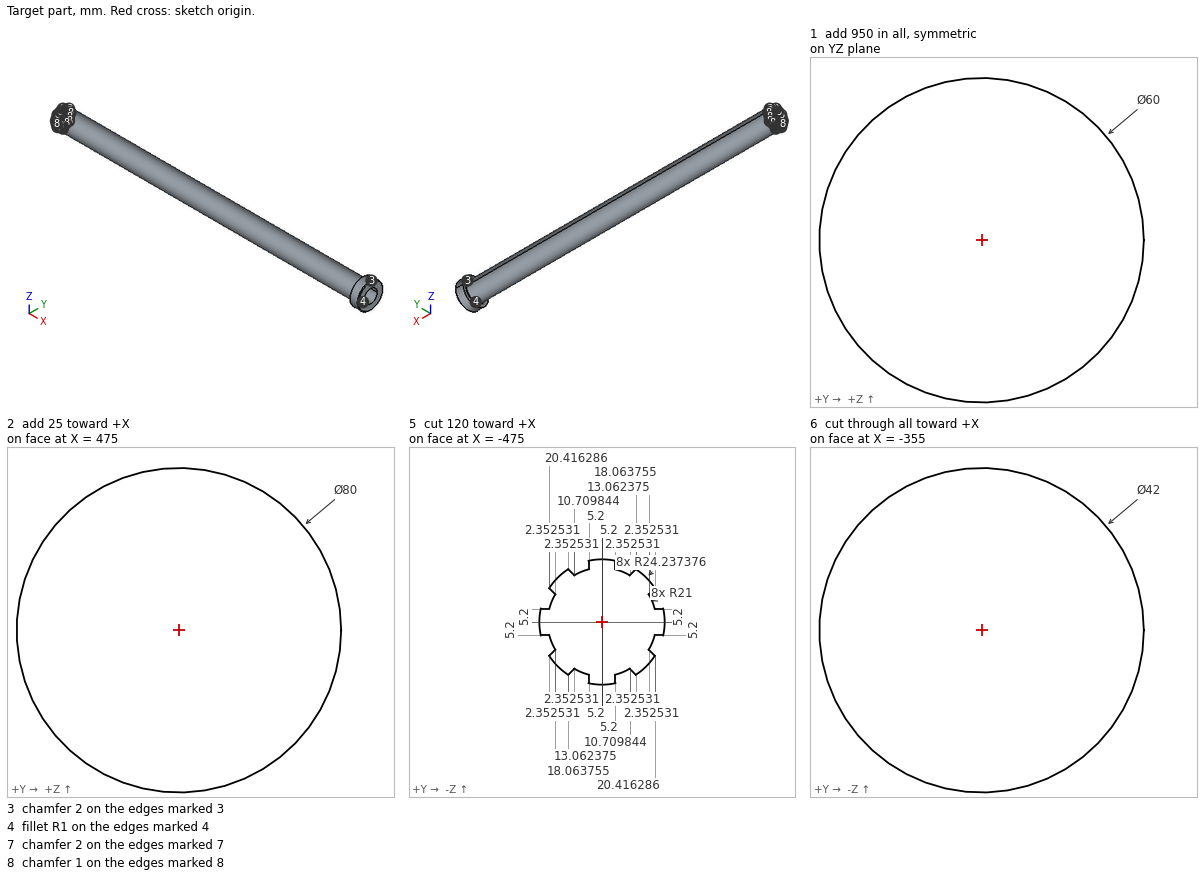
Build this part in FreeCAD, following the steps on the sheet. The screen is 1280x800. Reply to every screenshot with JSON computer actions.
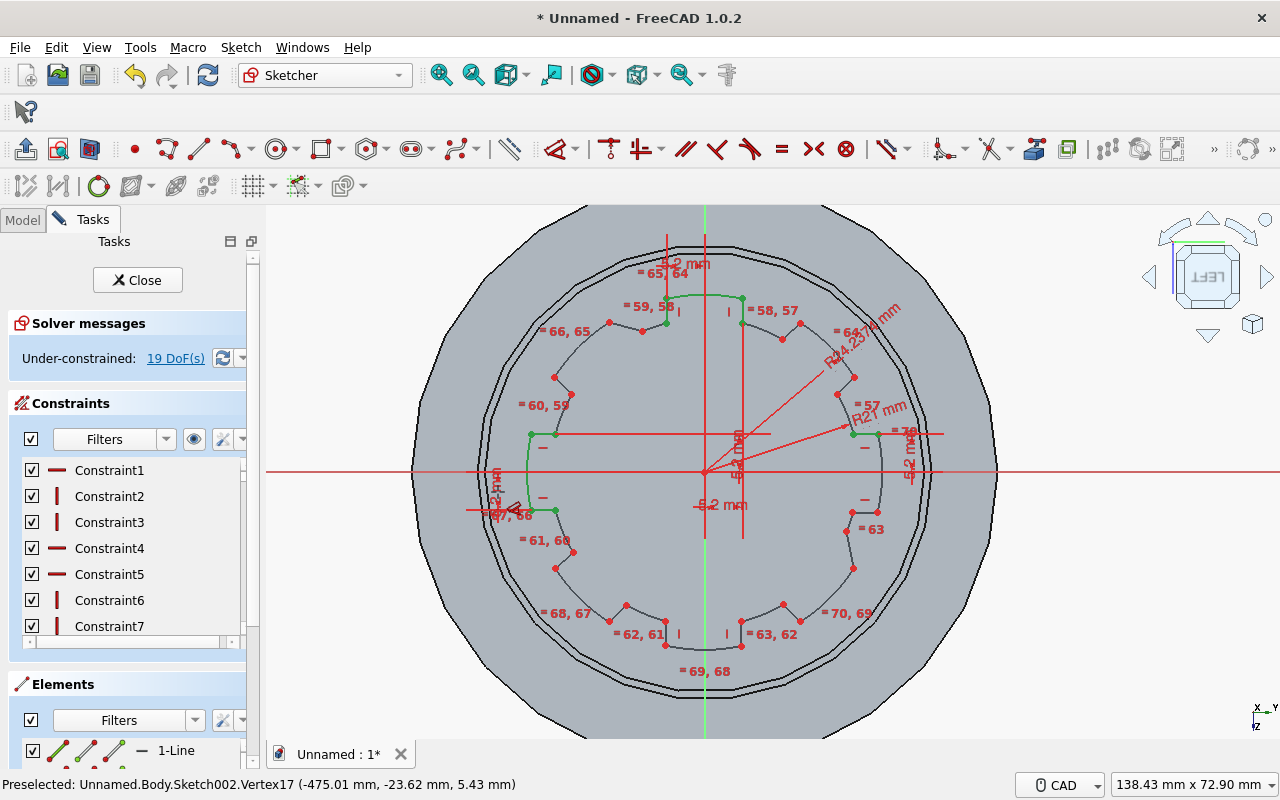
{"action": "left_click", "coordinate": [666, 621]}
{"action": "left_click", "coordinate": [685, 679]}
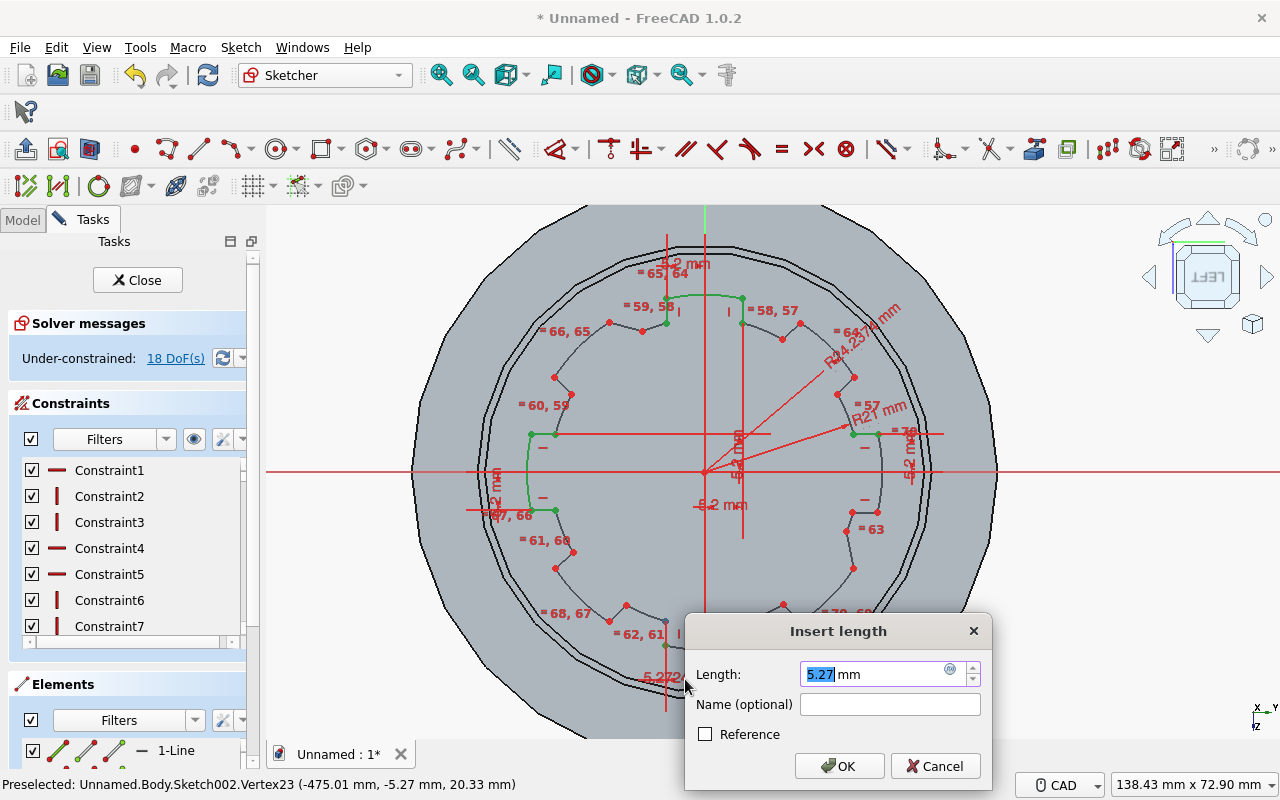
{"action": "type", "text": "5.2"}
{"action": "key", "text": "Return"}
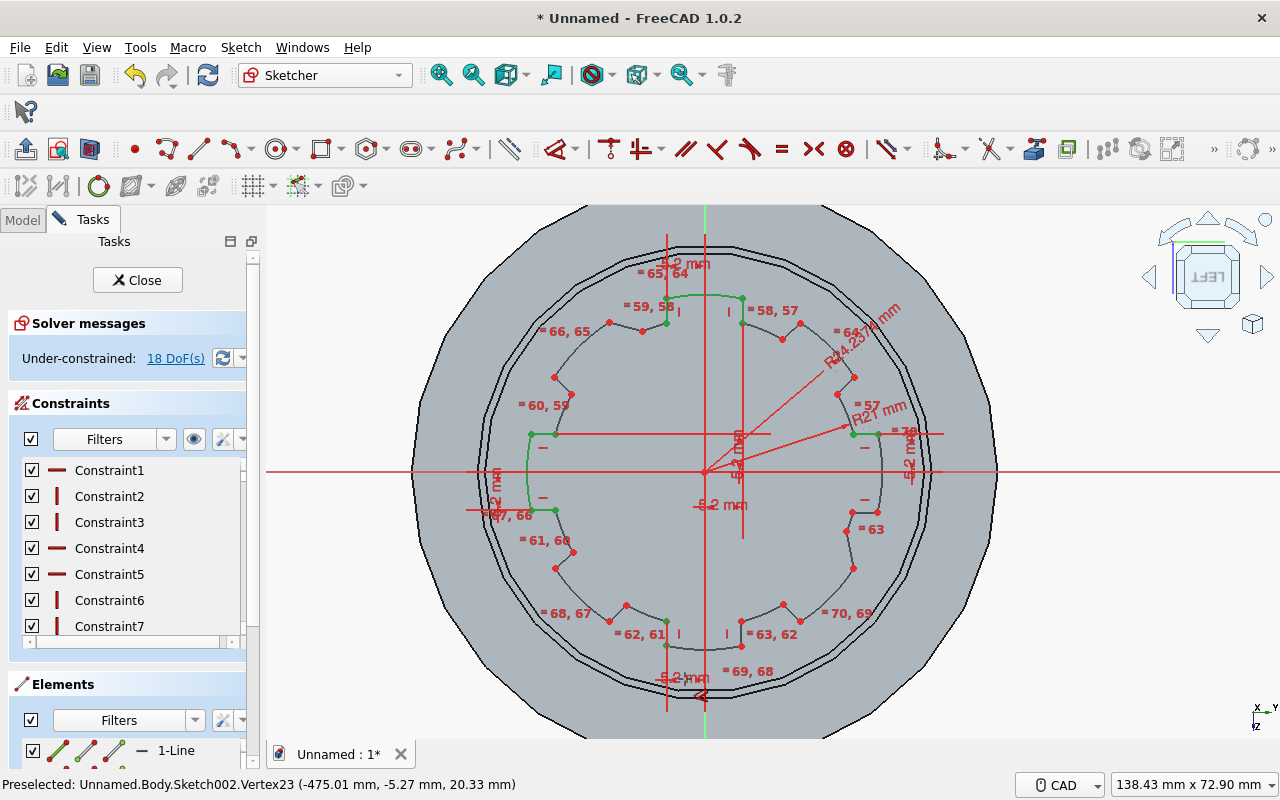
{"action": "left_click", "coordinate": [741, 646]}
{"action": "left_click", "coordinate": [723, 704]}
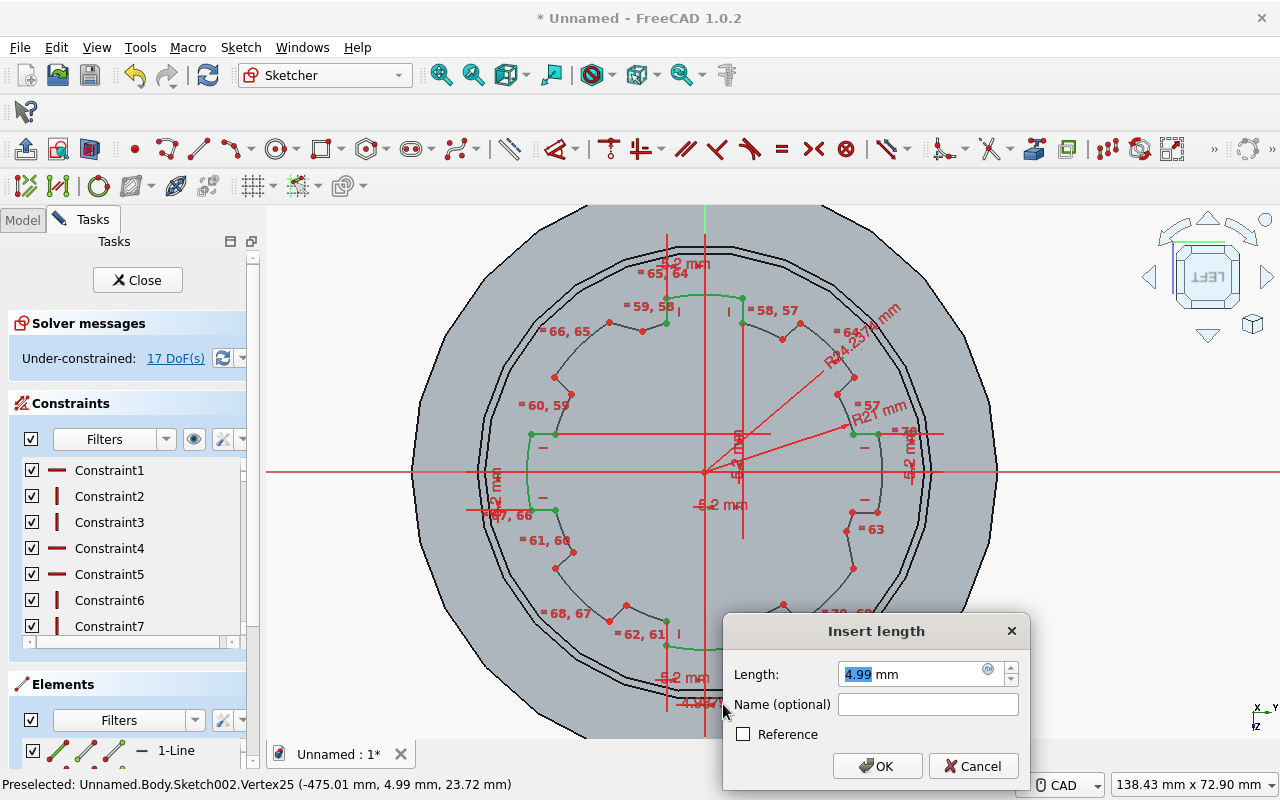
{"action": "type", "text": "5.2"}
{"action": "key", "text": "Return"}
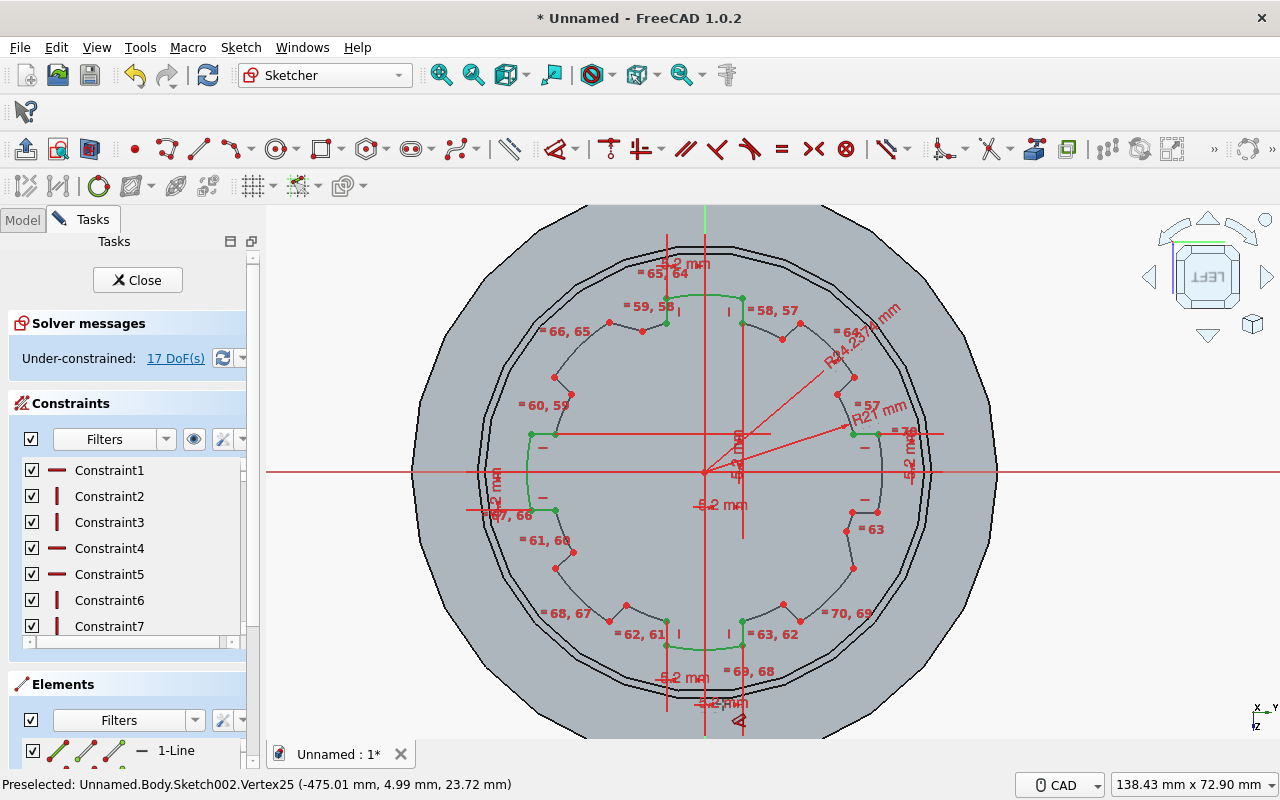
{"action": "left_click", "coordinate": [853, 513]}
{"action": "left_click", "coordinate": [911, 493]}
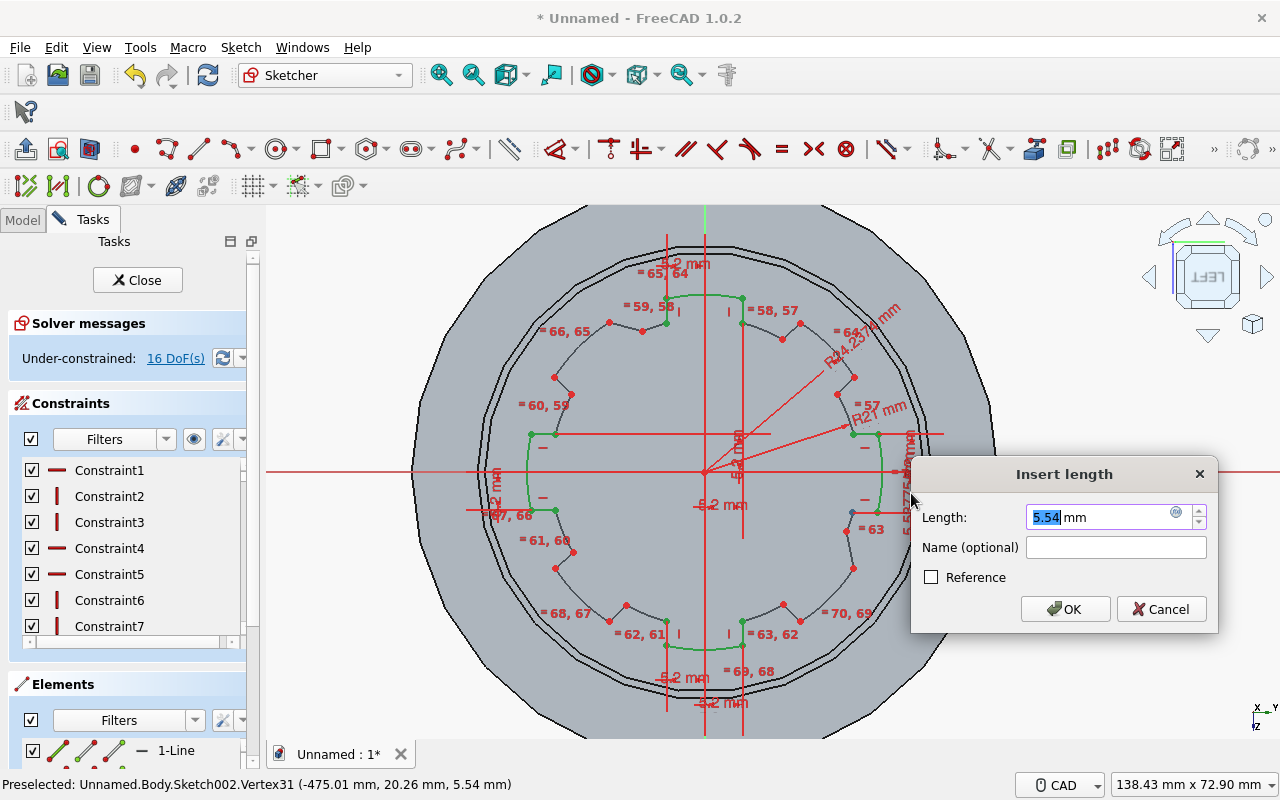
{"action": "type", "text": "5.2"}
{"action": "key", "text": "Return"}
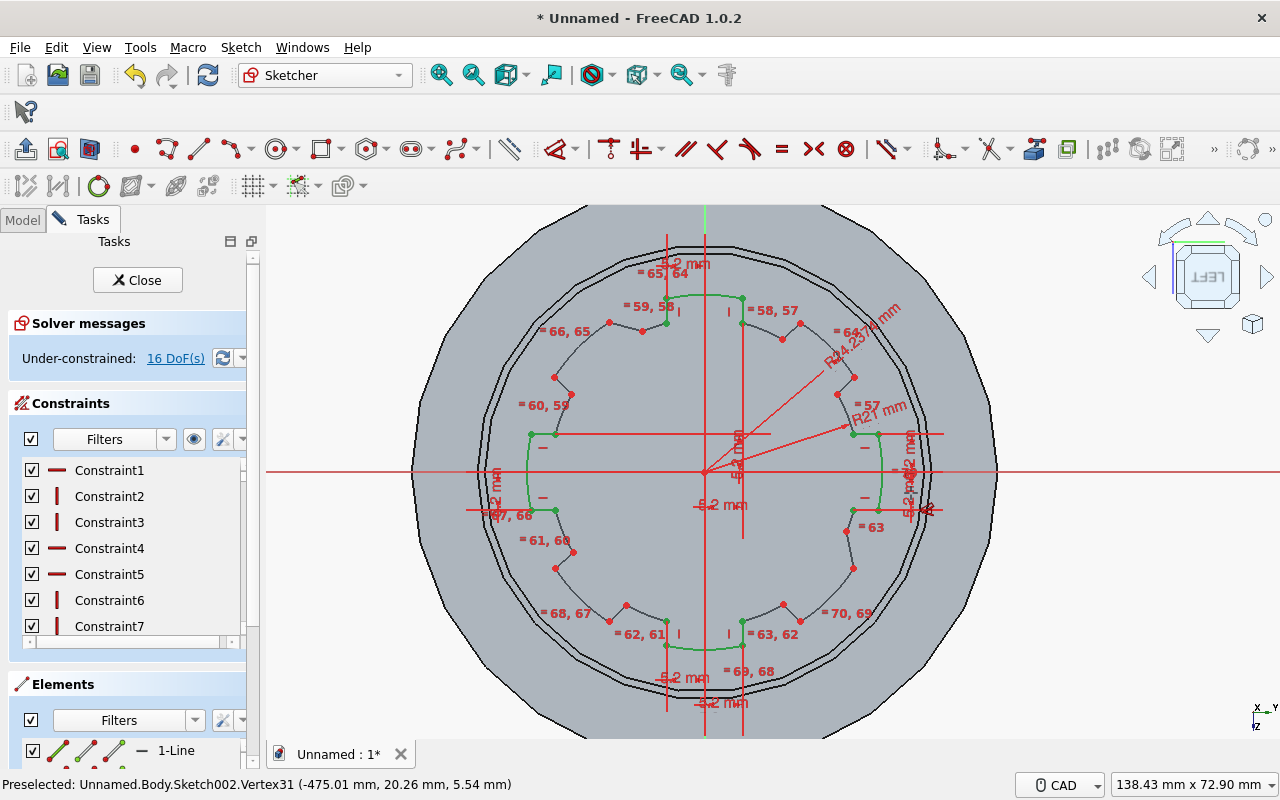
{"action": "scroll", "coordinate": [844, 388], "scroll_direction": "up", "scroll_amount": 5}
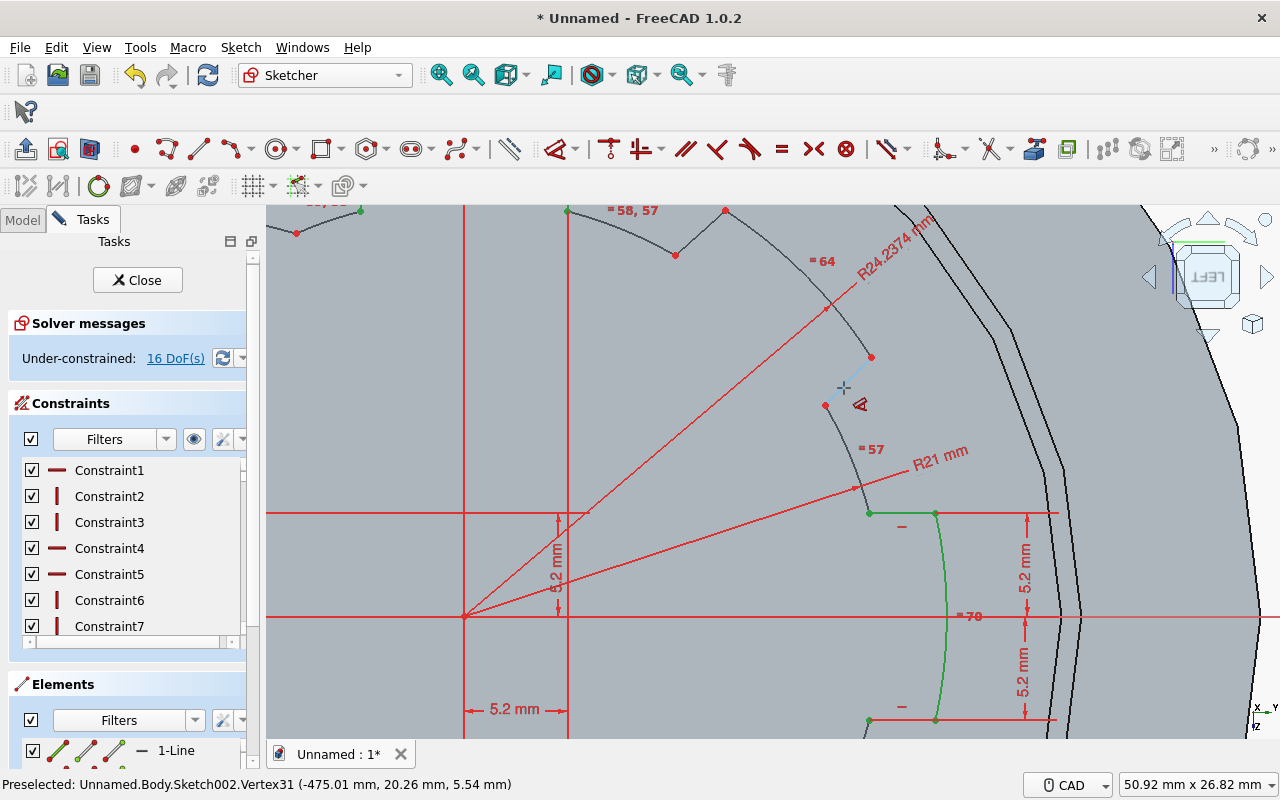
{"action": "left_click", "coordinate": [844, 386]}
{"action": "left_click", "coordinate": [865, 324]}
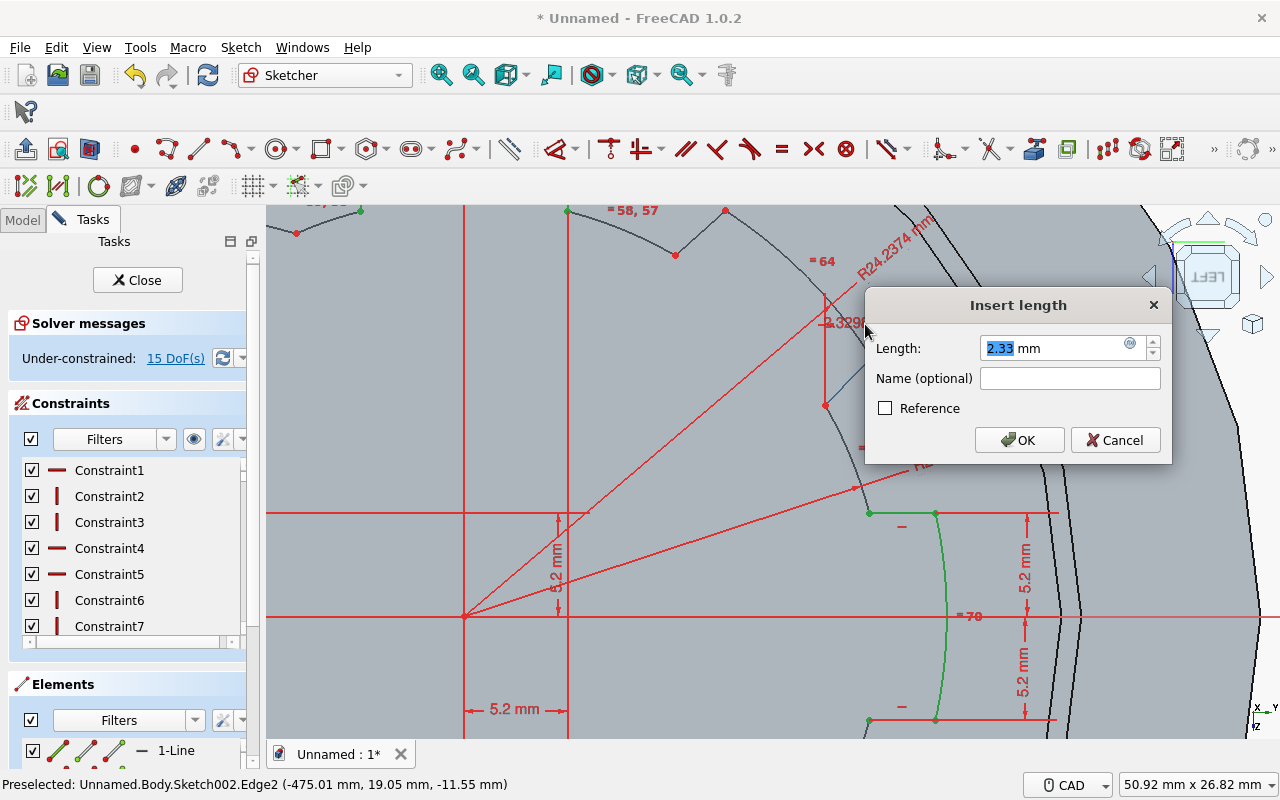
{"action": "type", "text": "2.352531"}
{"action": "key", "text": "Return"}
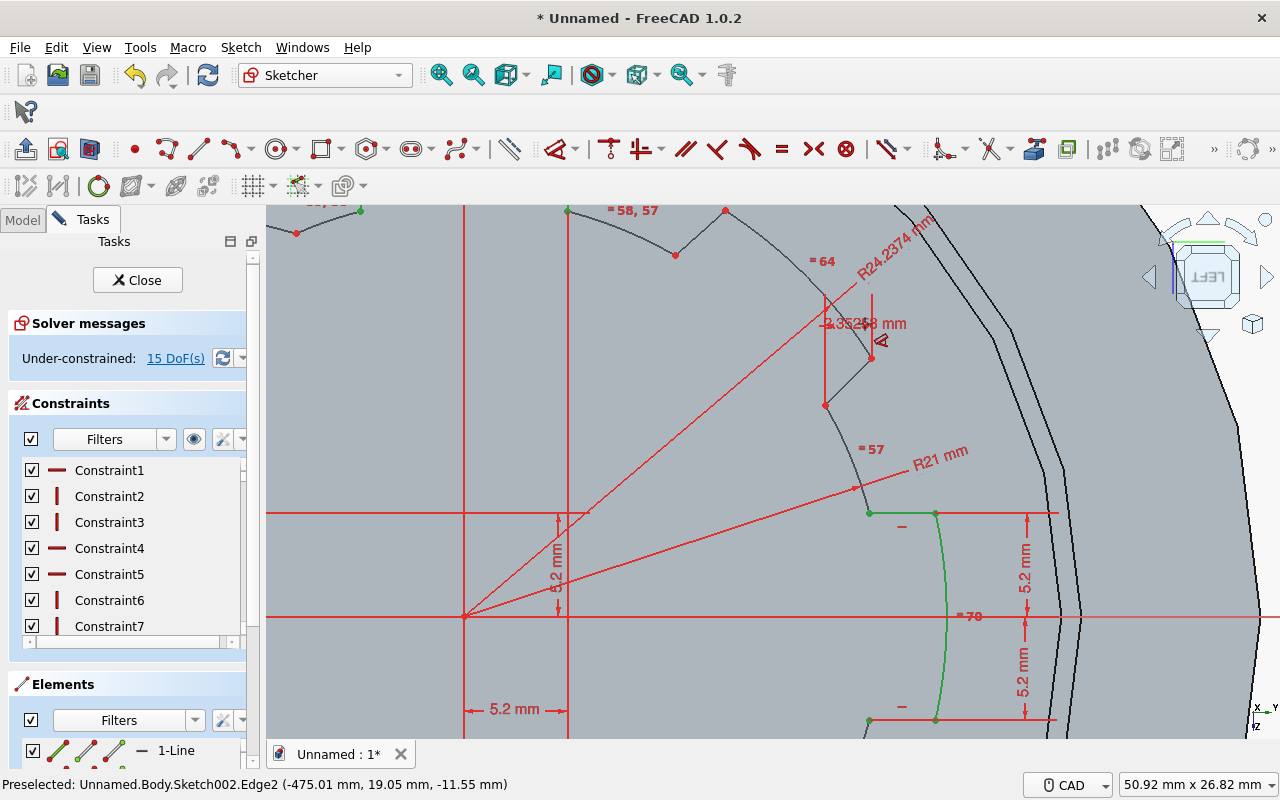
{"action": "left_click", "coordinate": [690, 242]}
{"action": "left_click", "coordinate": [700, 290]}